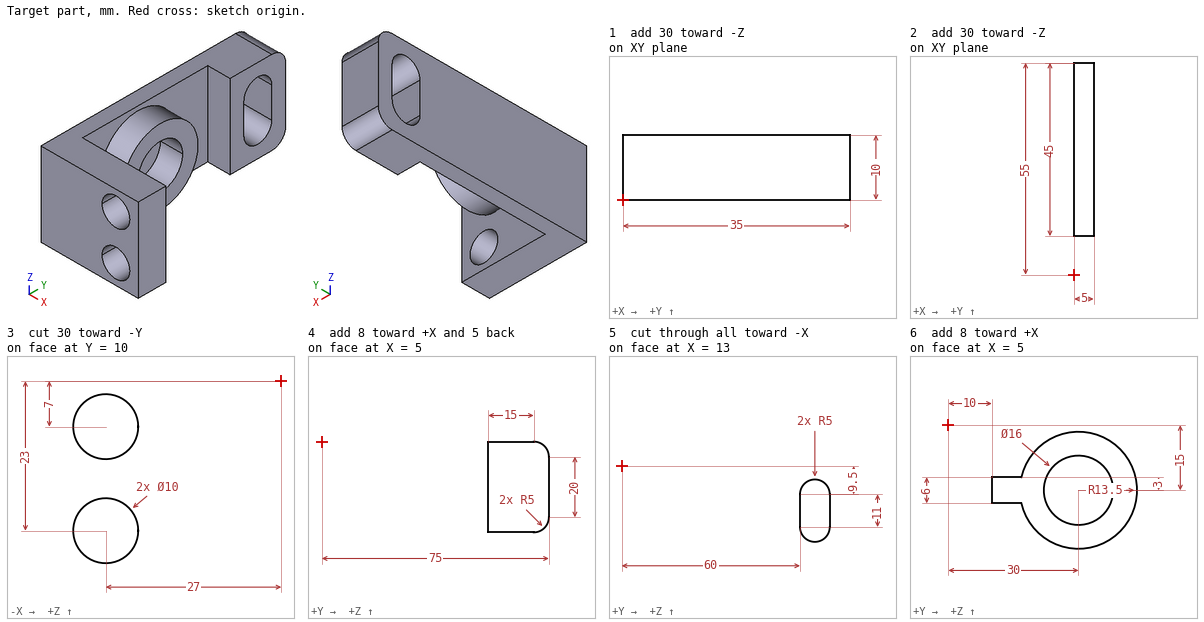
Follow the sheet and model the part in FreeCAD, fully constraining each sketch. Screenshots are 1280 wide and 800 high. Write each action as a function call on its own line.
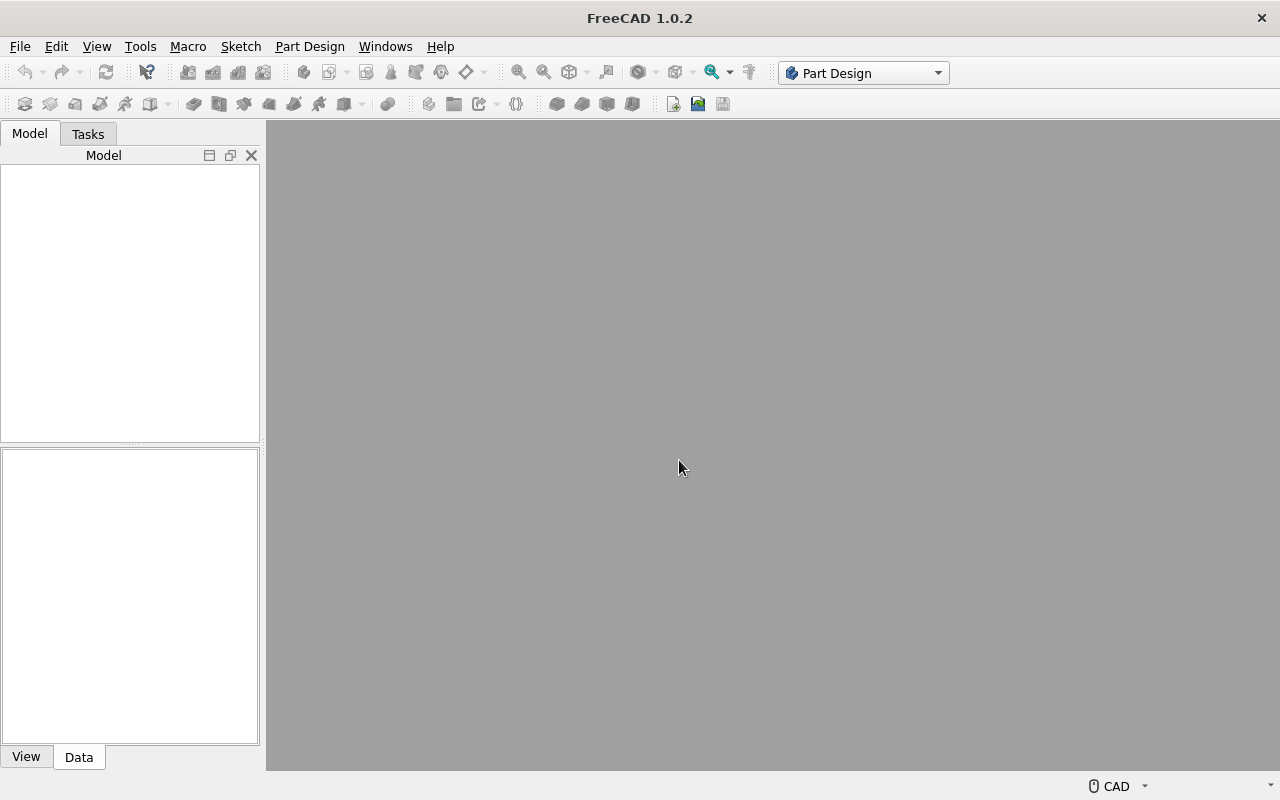
key(ctrl+n)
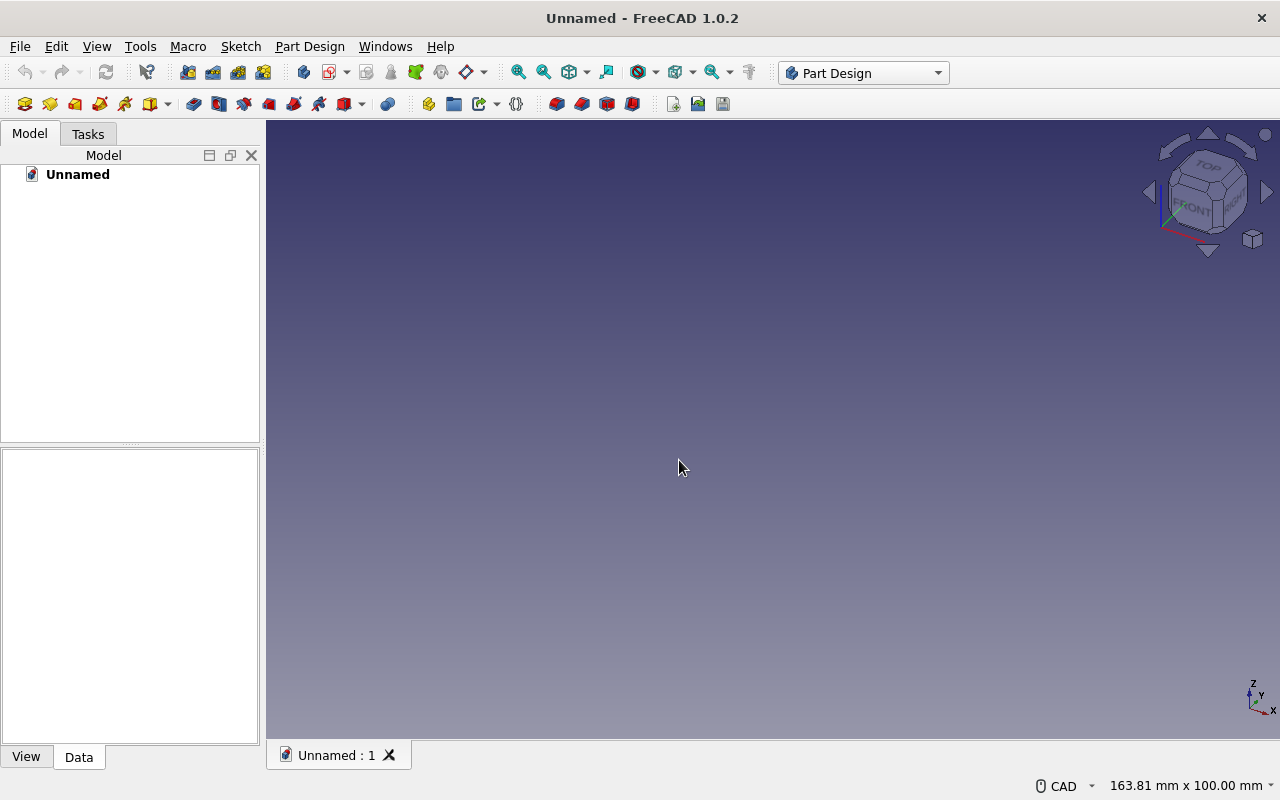
click(328, 72)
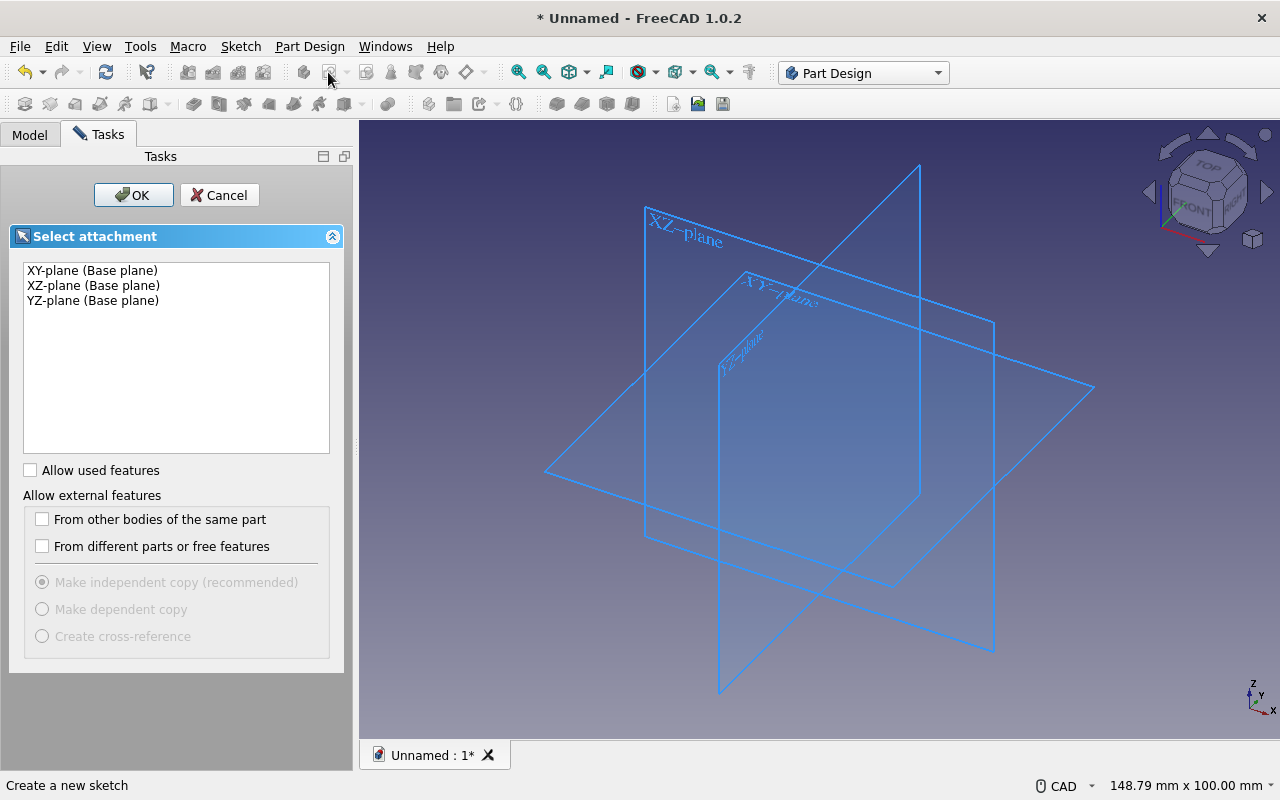
click(84, 270)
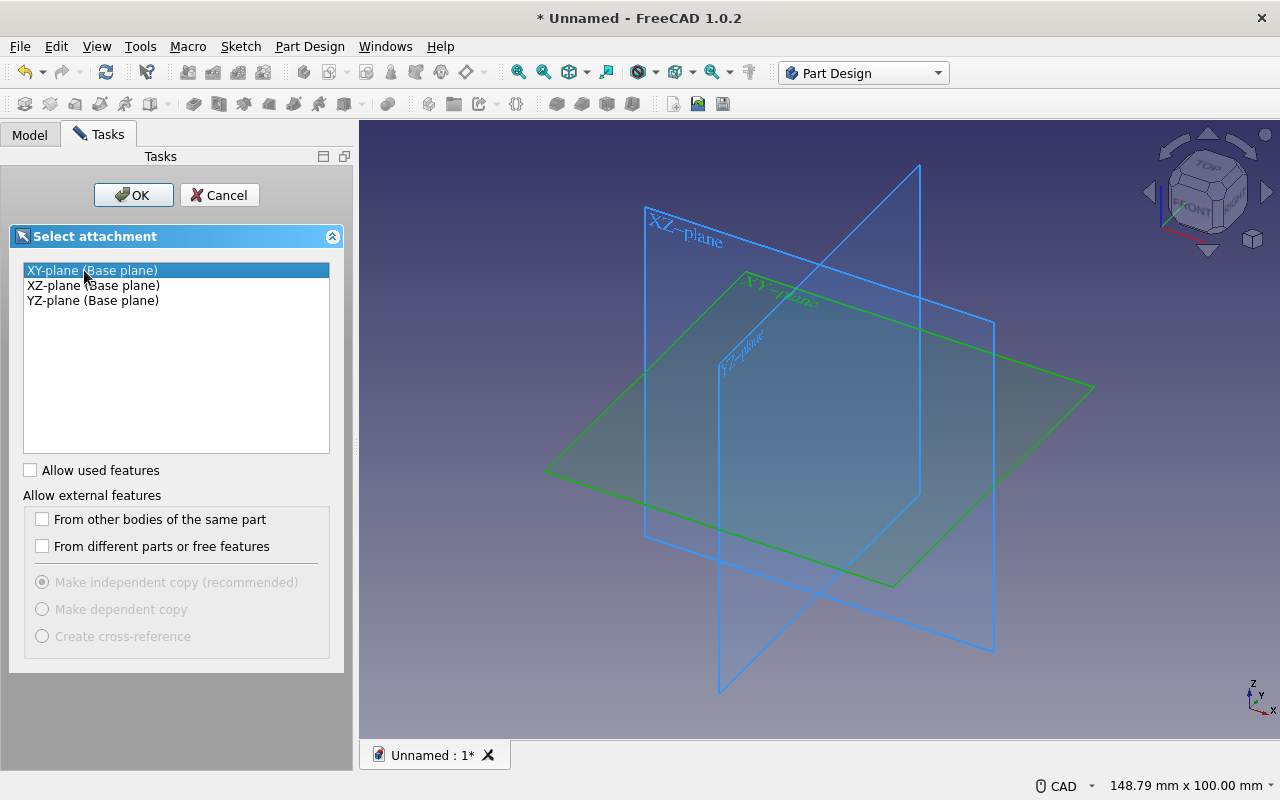
click(134, 195)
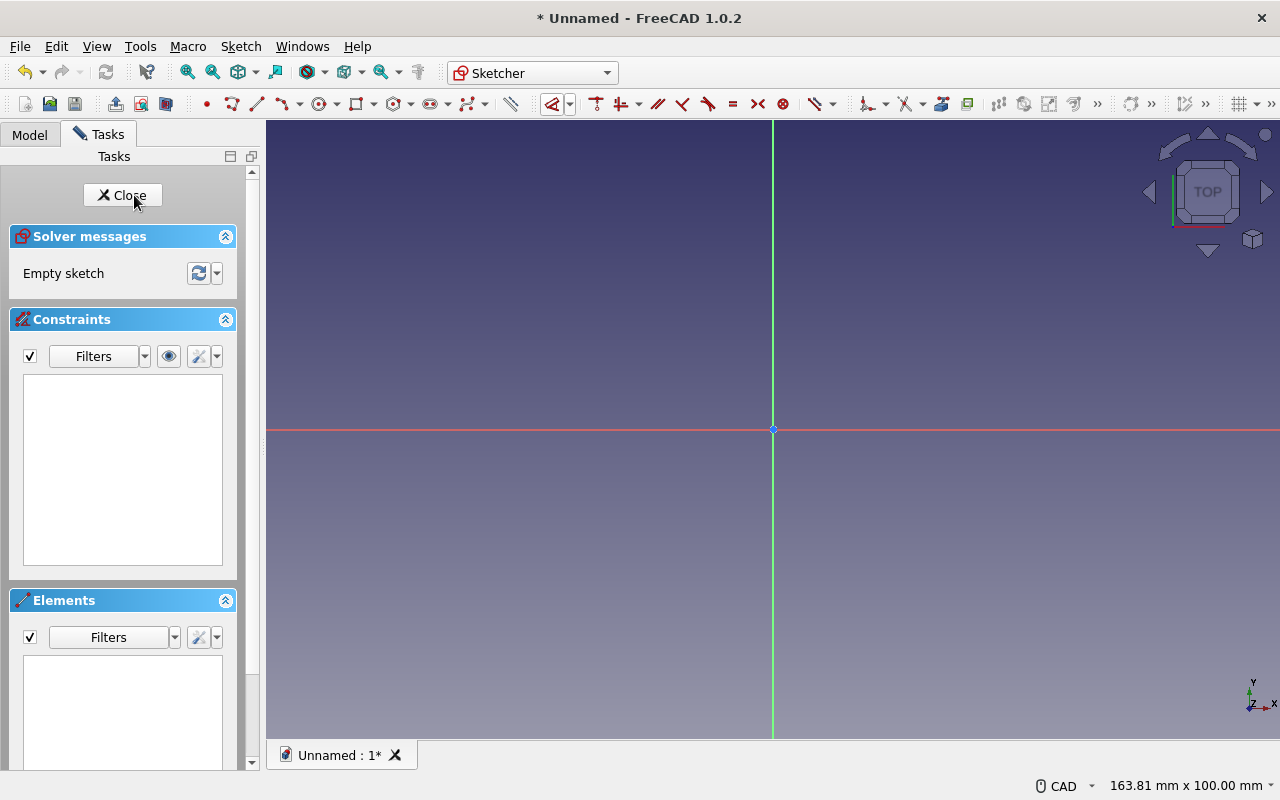
scroll(984, 381, up, 5)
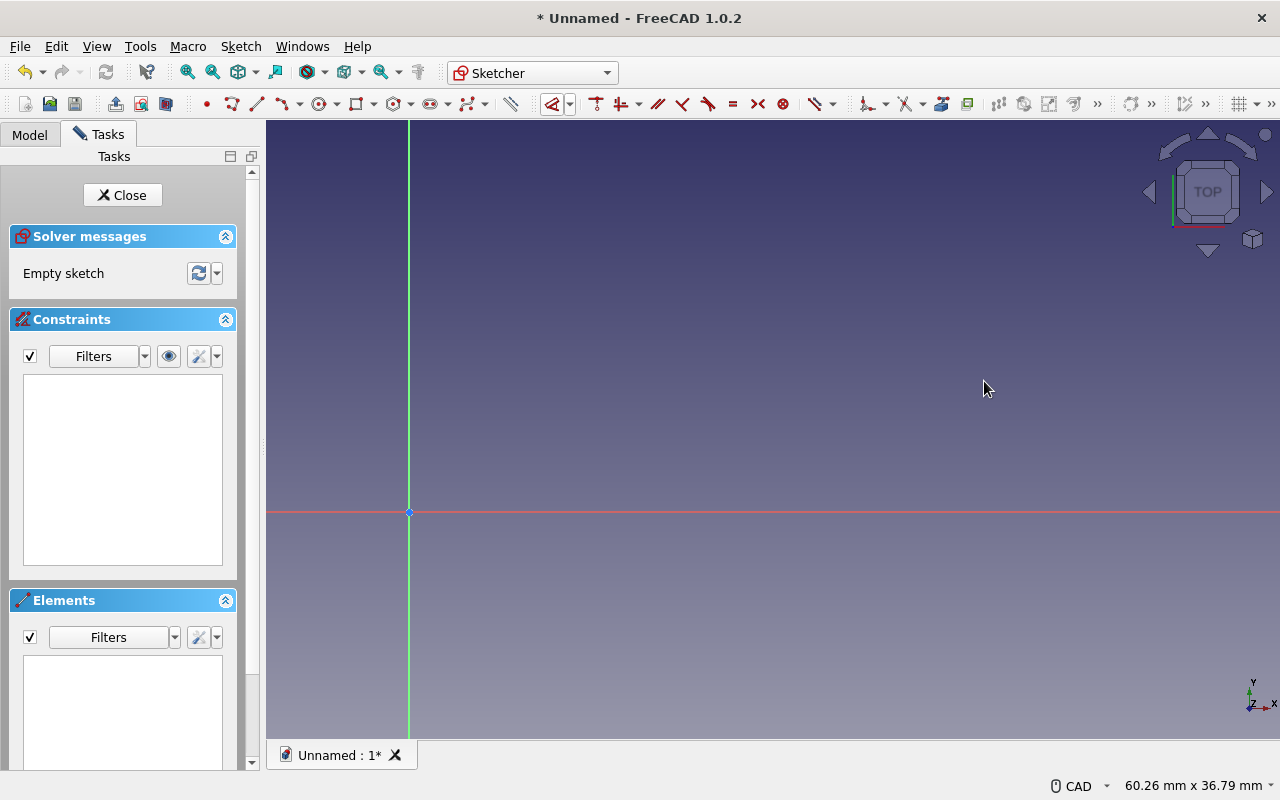
key(g)
key(r)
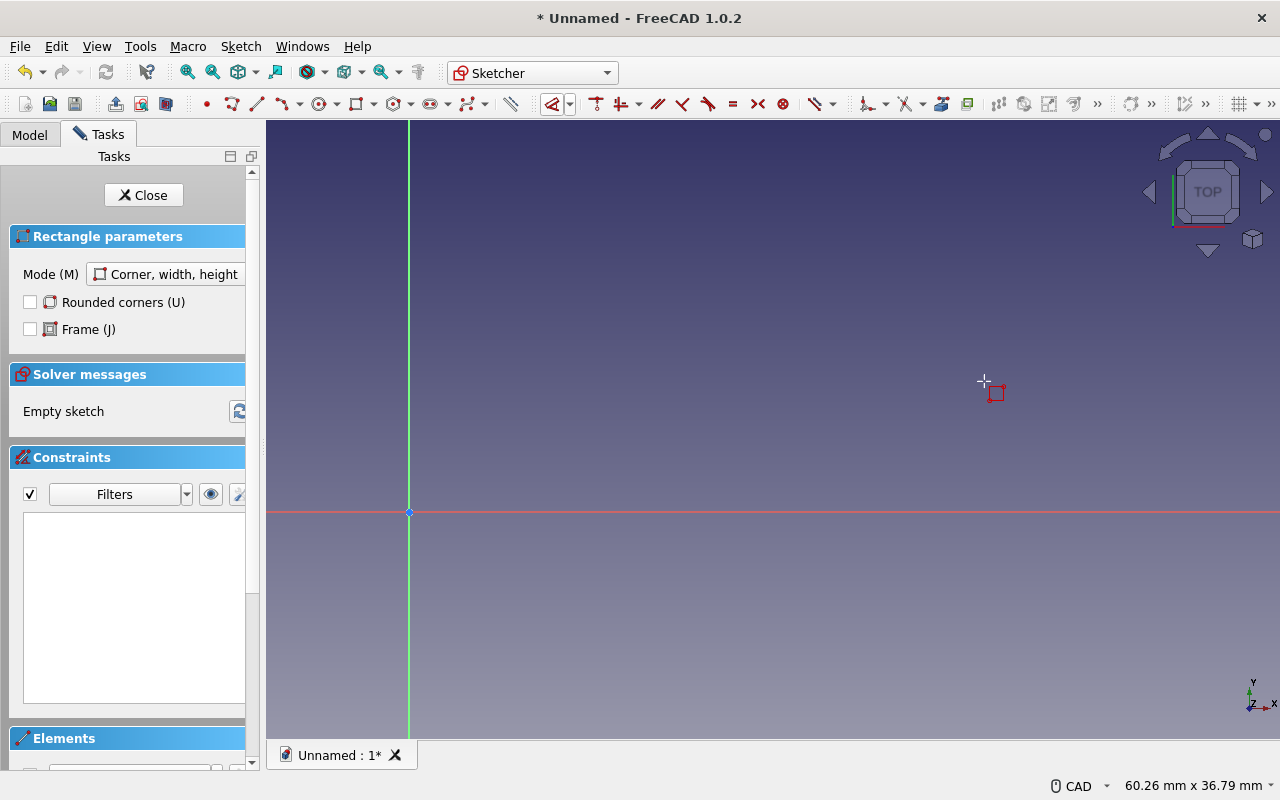
click(409, 512)
click(998, 344)
key(Escape)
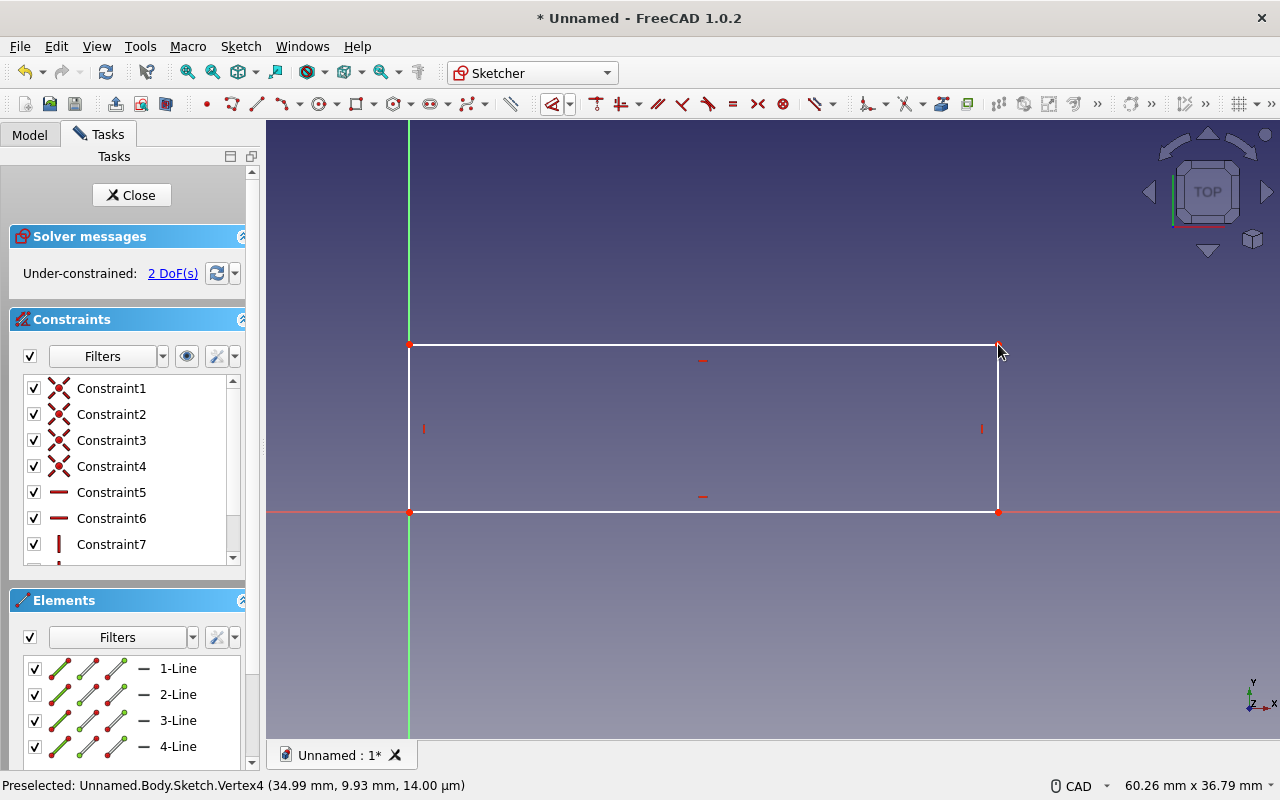
key(d)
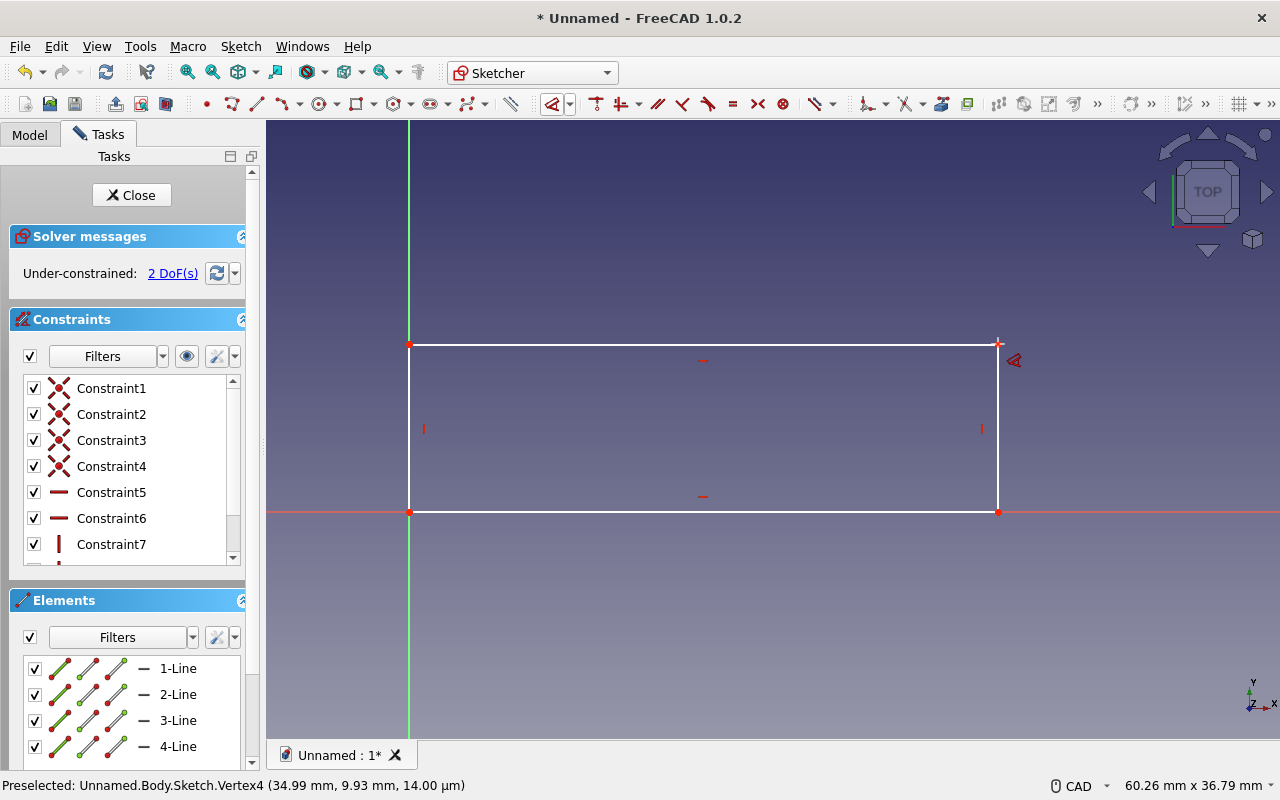
click(586, 512)
click(704, 546)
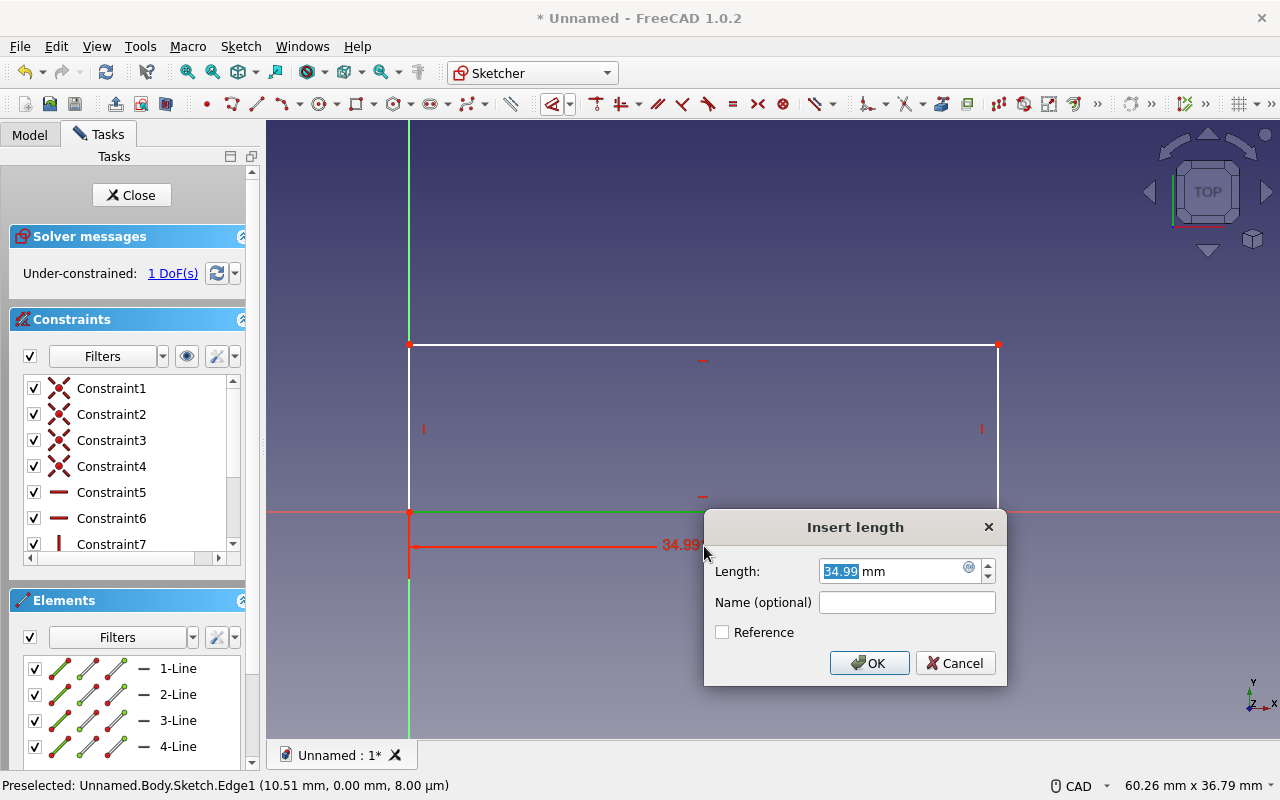
text(35)
key(Return)